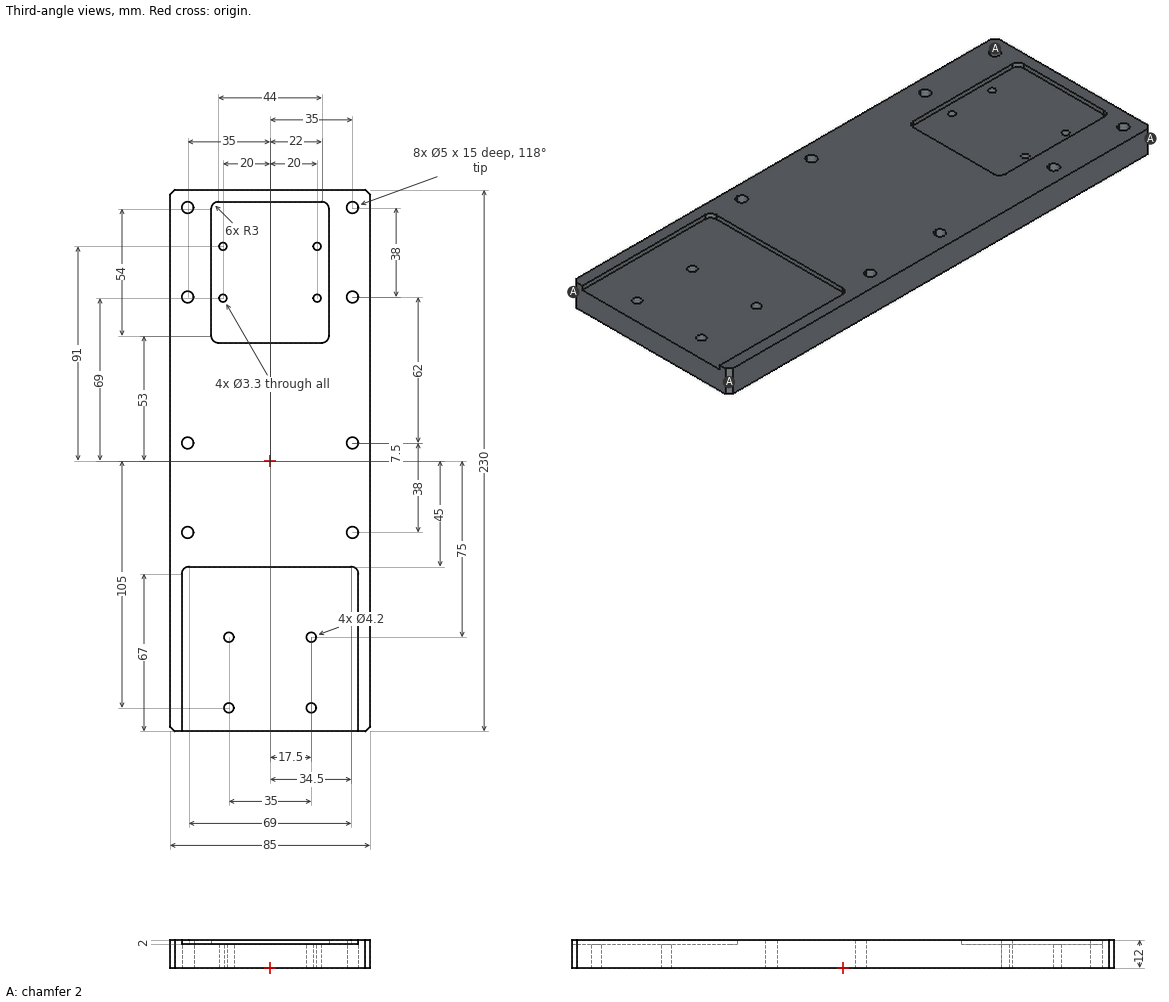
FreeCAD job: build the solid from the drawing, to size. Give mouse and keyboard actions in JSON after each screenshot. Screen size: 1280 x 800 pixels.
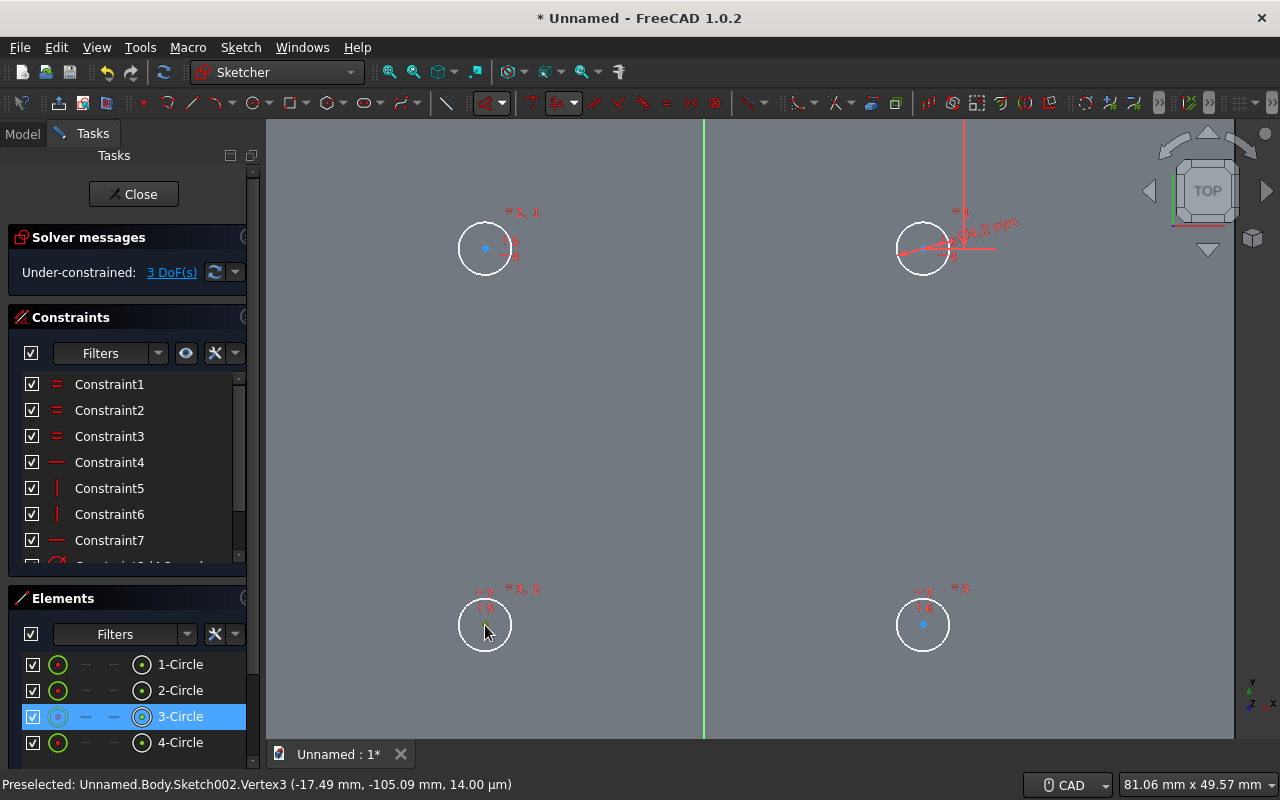
{"action": "key", "text": "i"}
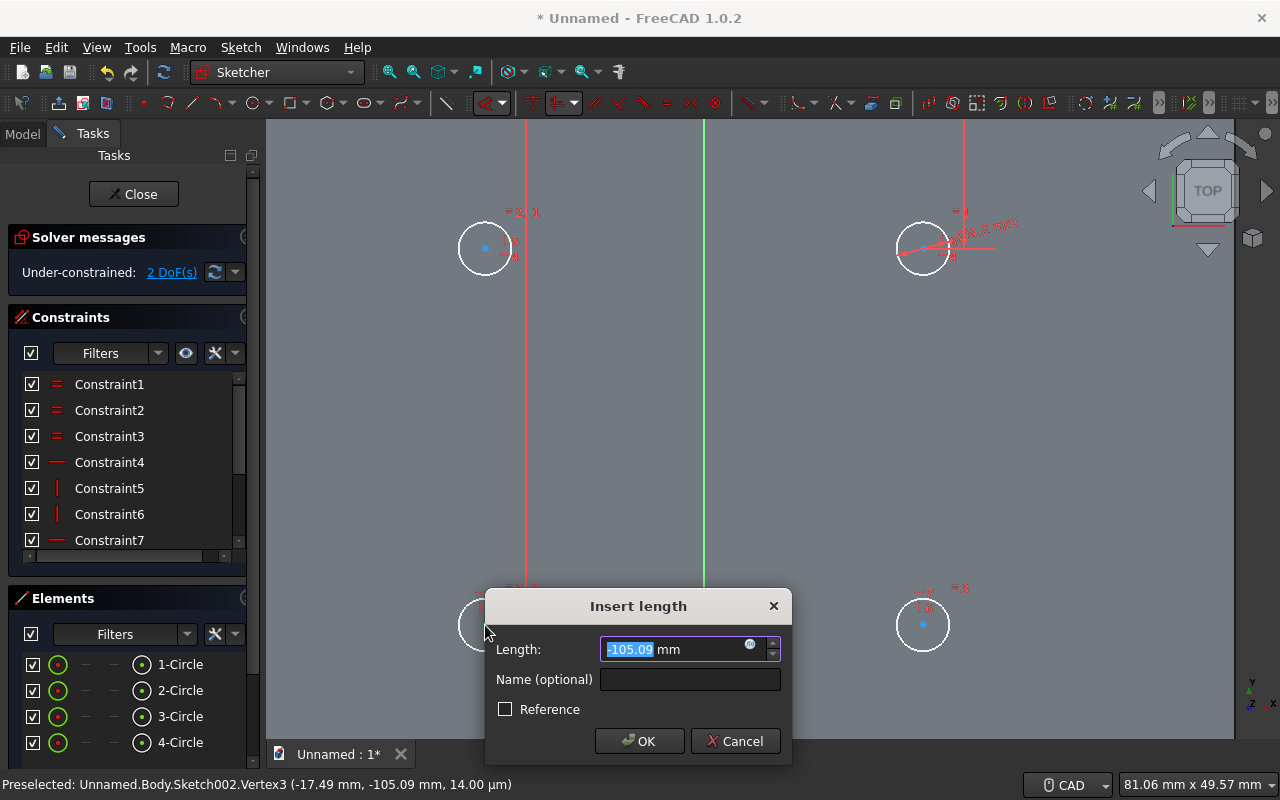
{"action": "type", "text": "-105"}
{"action": "key", "text": "Return"}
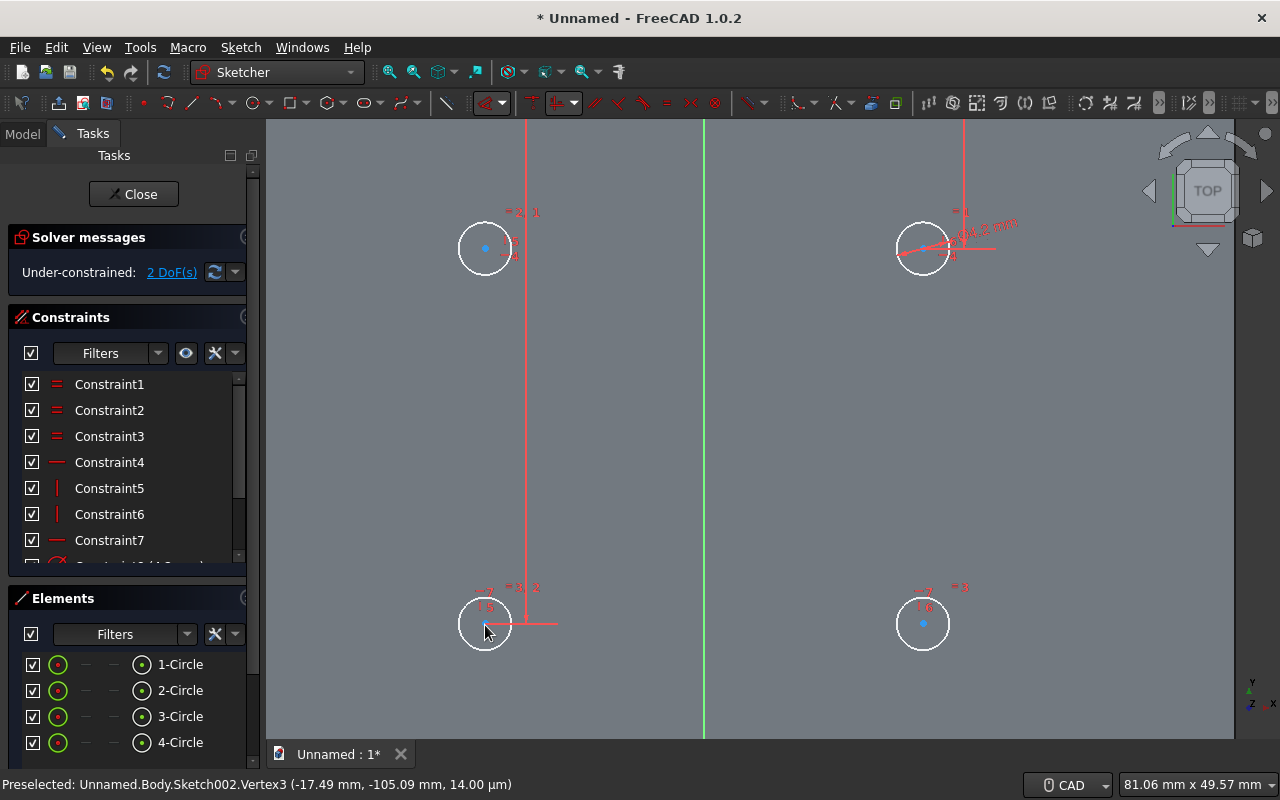
{"action": "left_click", "coordinate": [923, 249]}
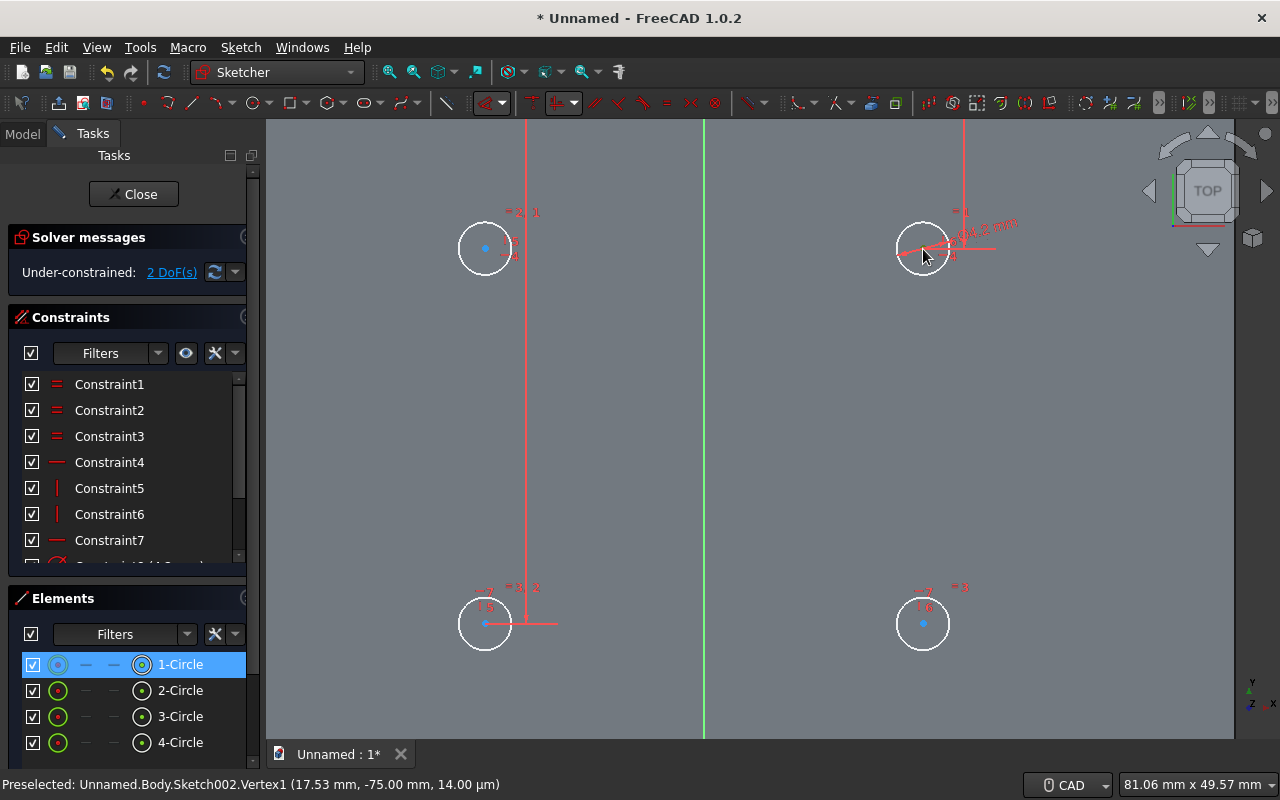
{"action": "left_click", "coordinate": [485, 249]}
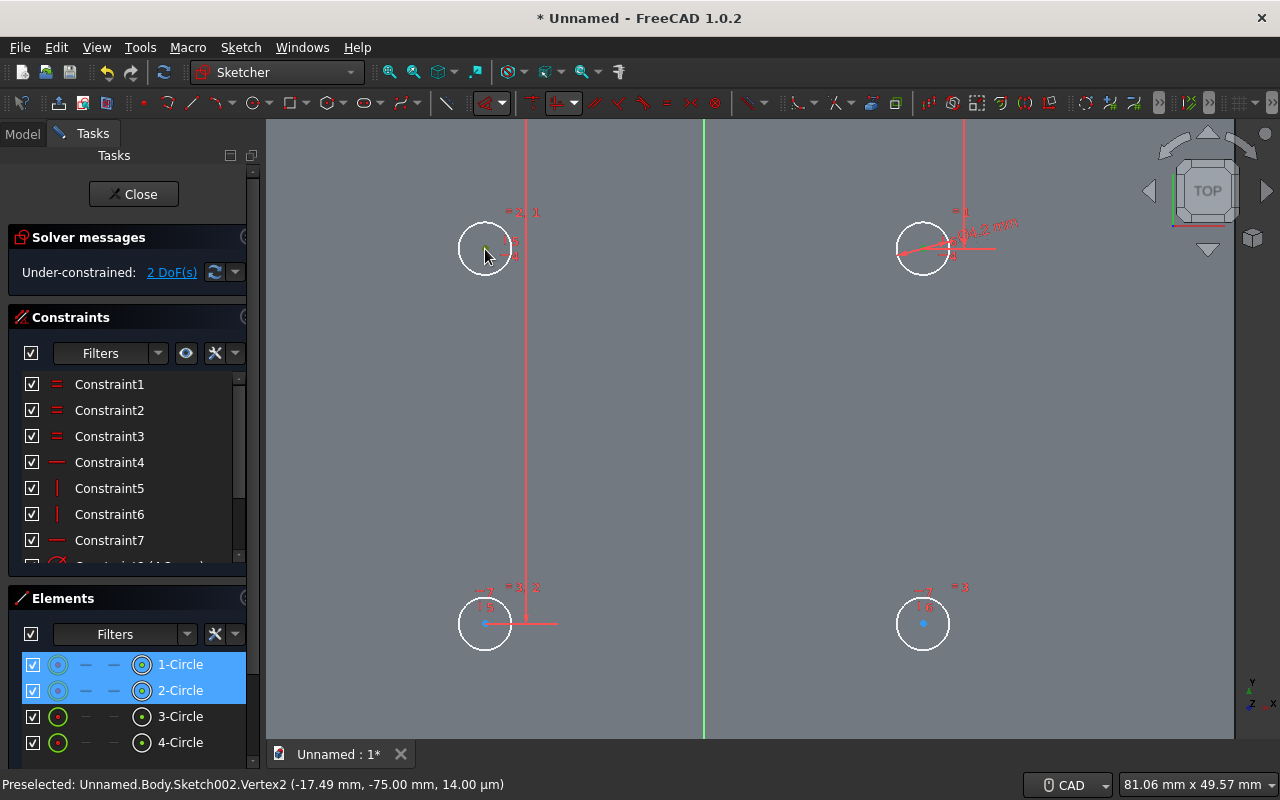
{"action": "key", "text": "l"}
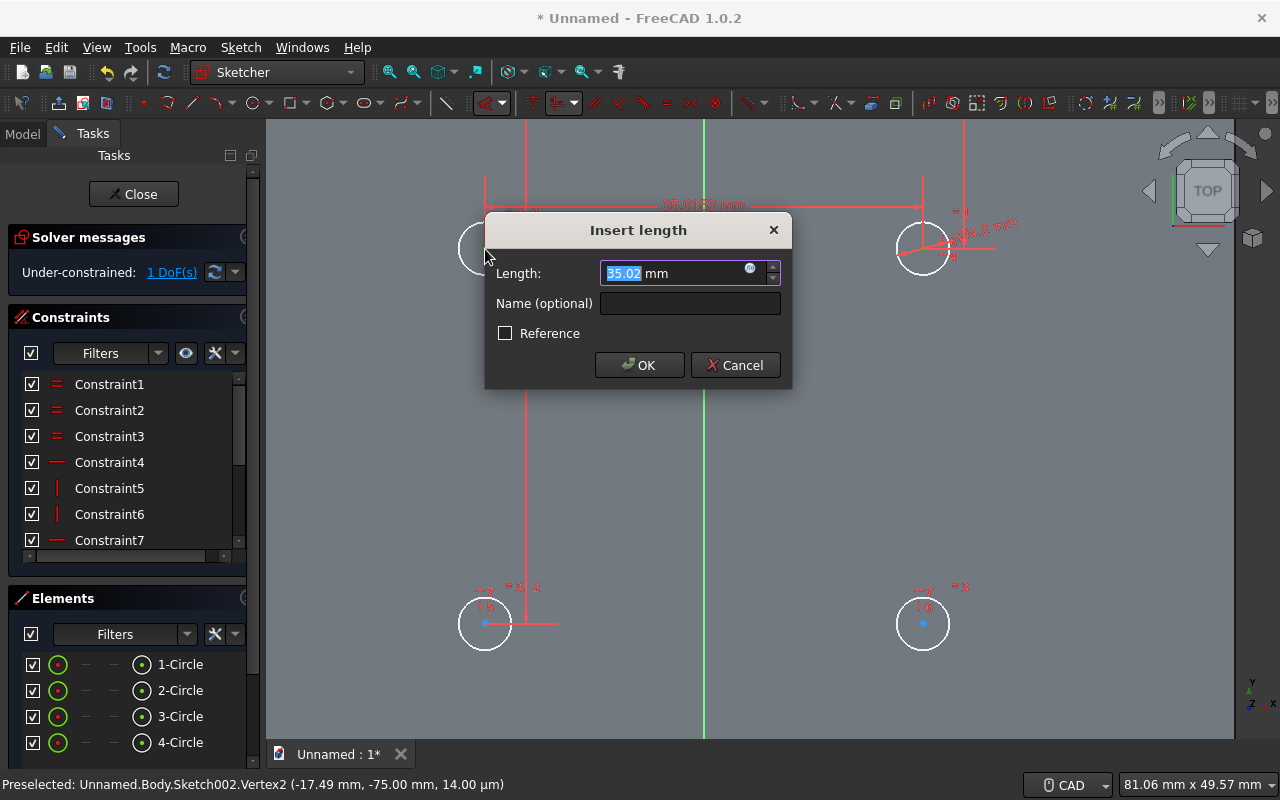
{"action": "type", "text": "35"}
{"action": "key", "text": "Return"}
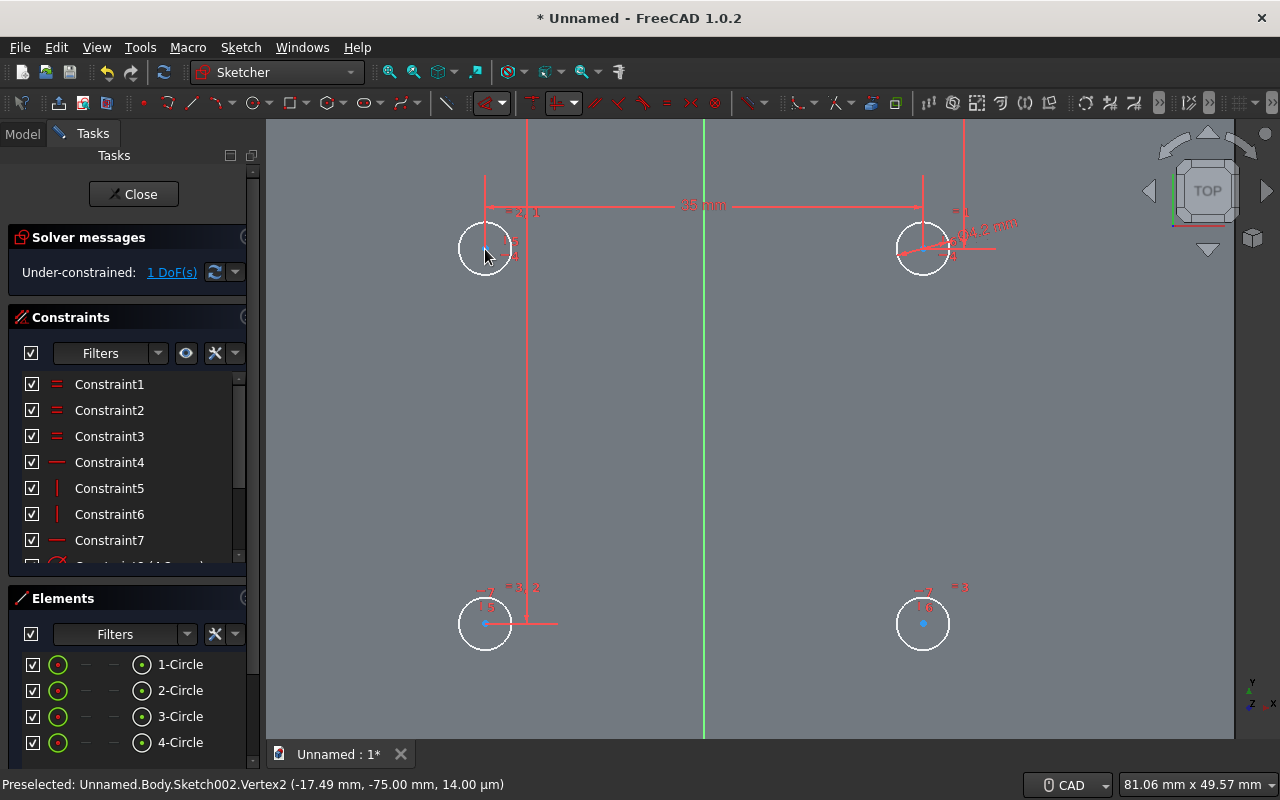
{"action": "left_click", "coordinate": [923, 249]}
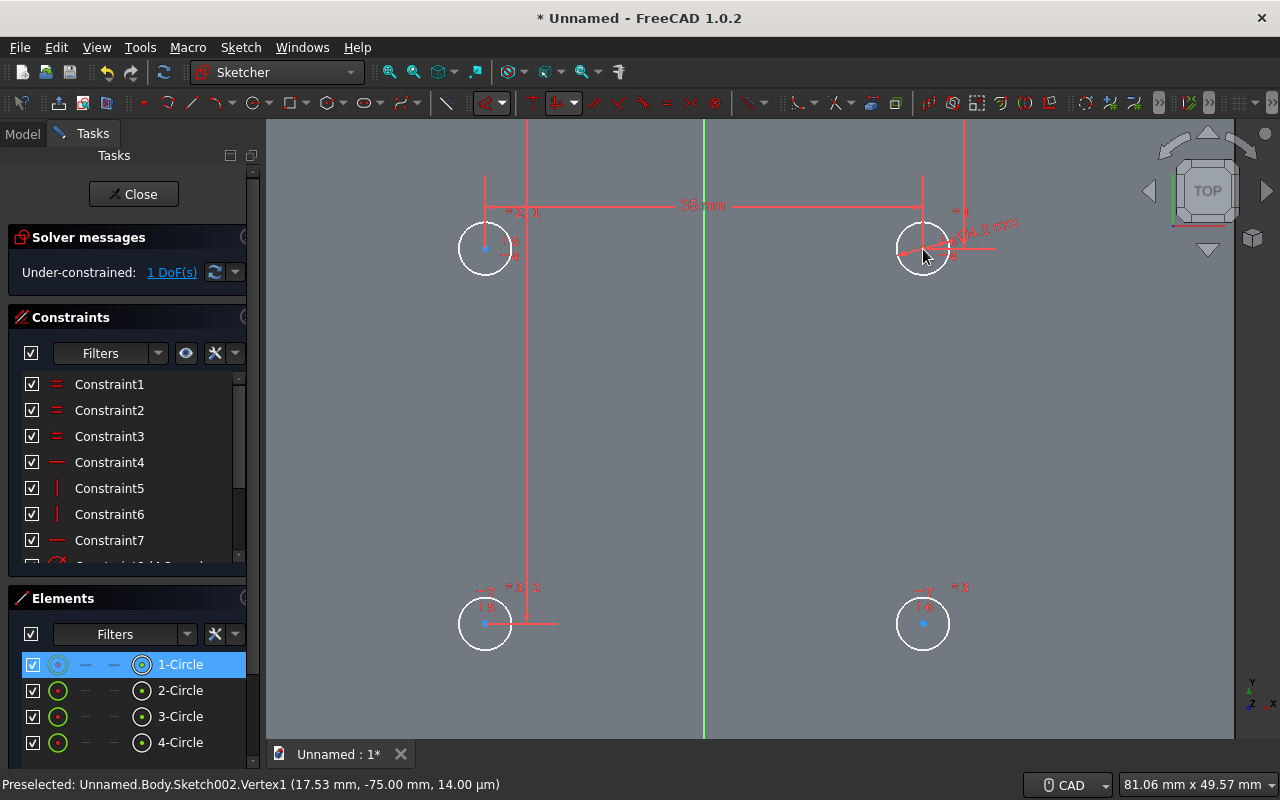
{"action": "key", "text": "l"}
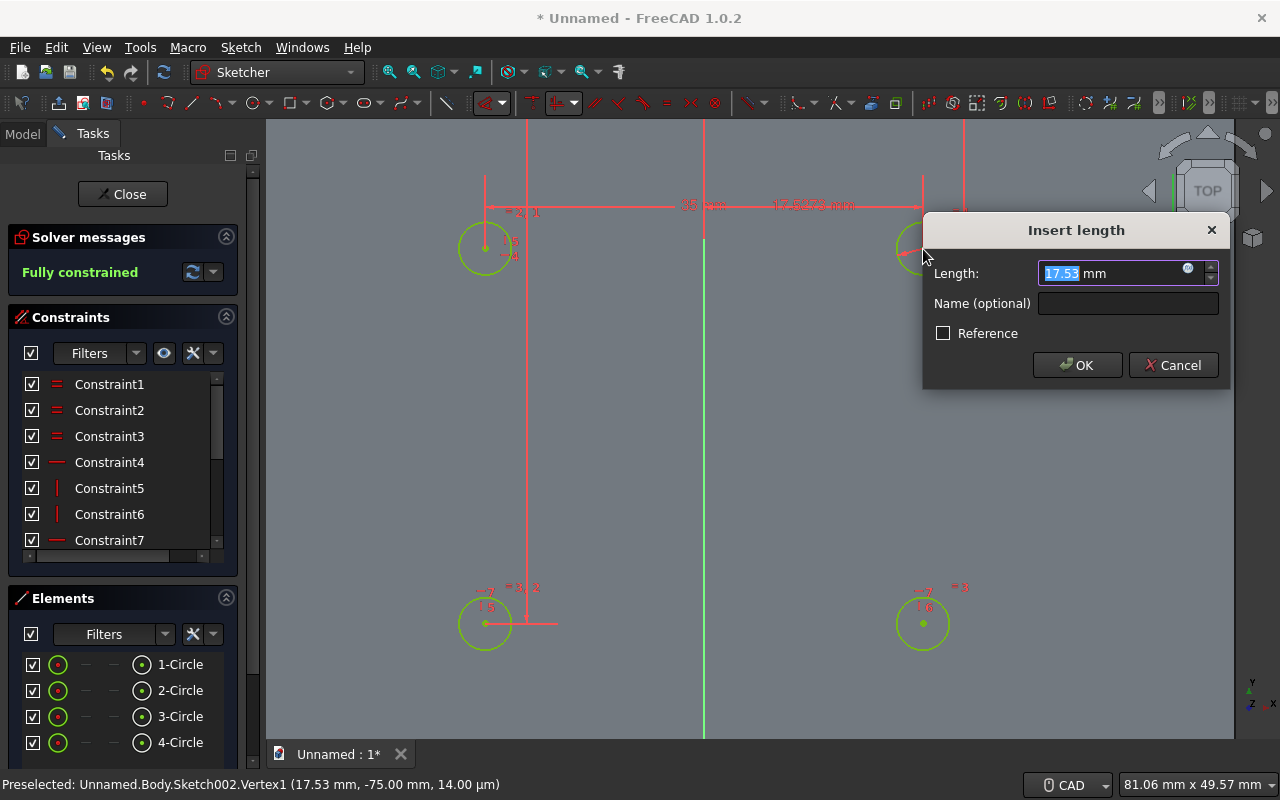
{"action": "type", "text": "17.5"}
{"action": "key", "text": "Return"}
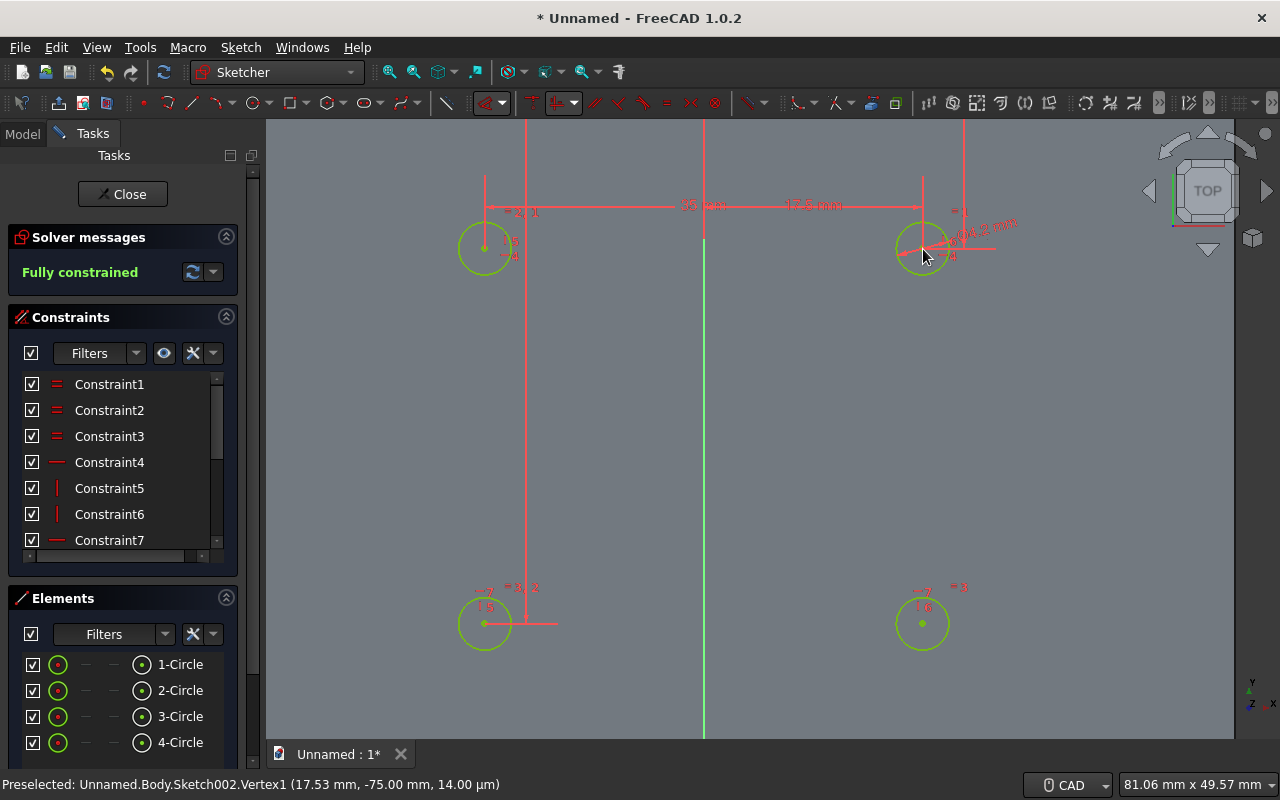
{"action": "left_click", "coordinate": [123, 194]}